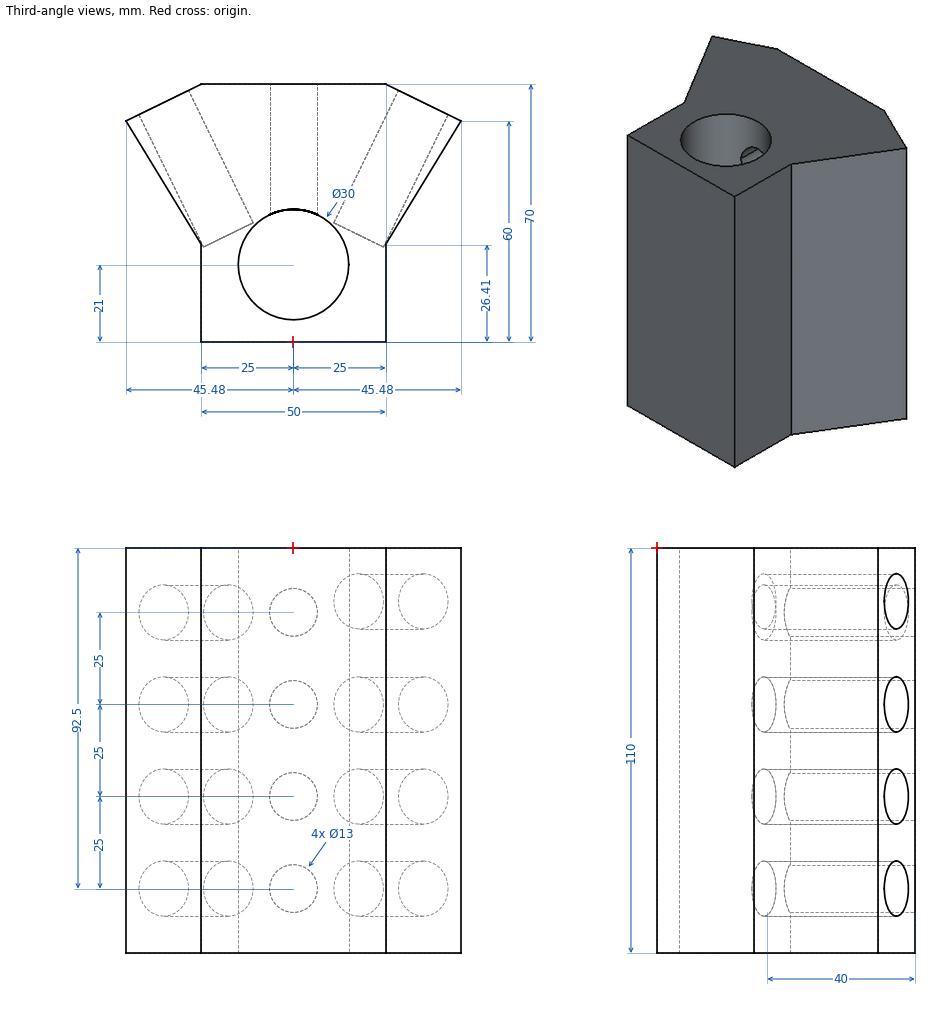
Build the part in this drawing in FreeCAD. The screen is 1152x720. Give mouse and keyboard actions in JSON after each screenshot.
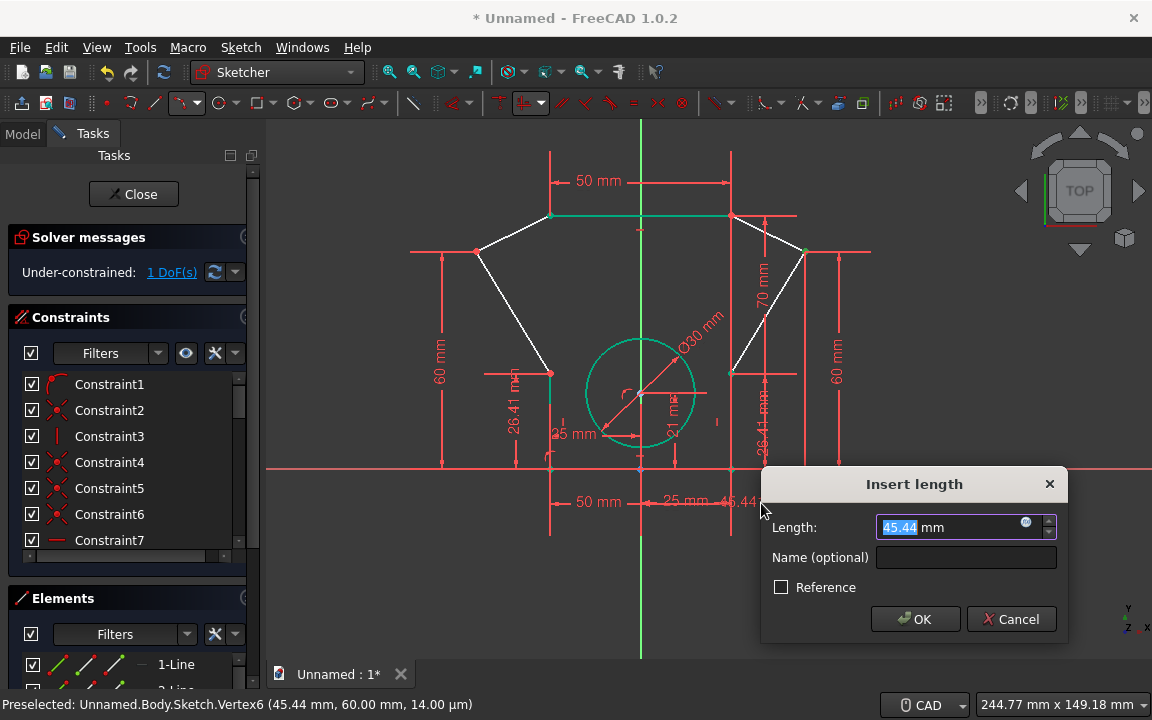
{"action": "type", "text": "45.48"}
{"action": "key", "text": "Return"}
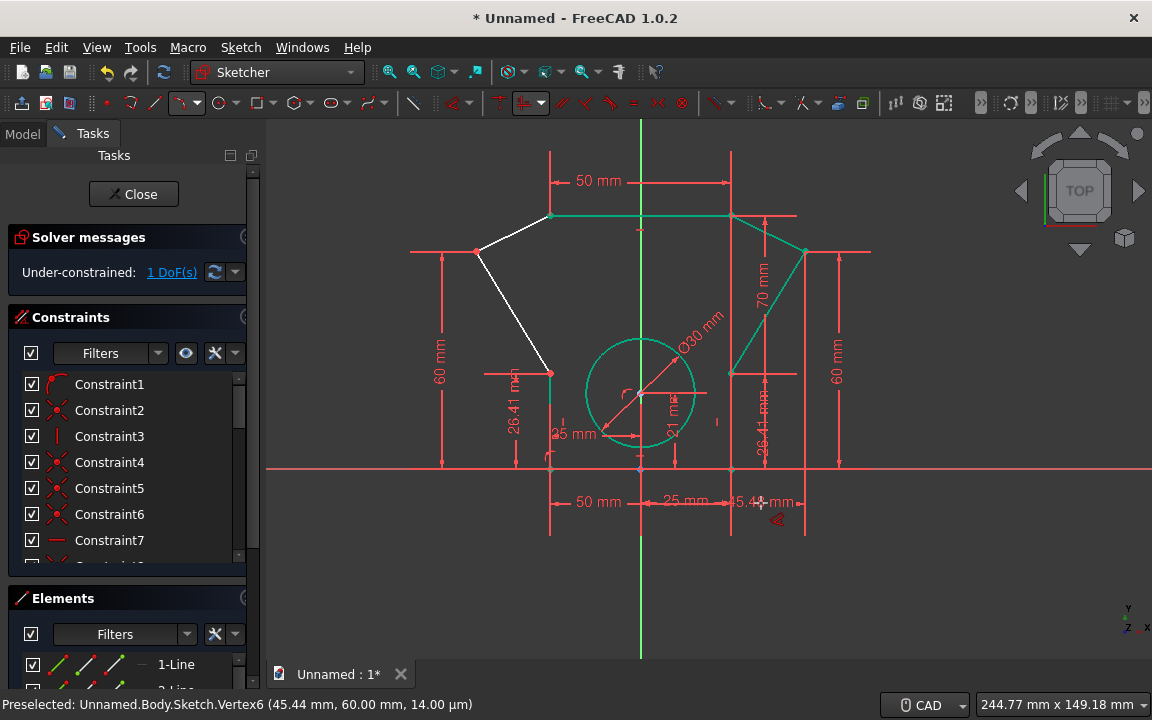
{"action": "left_click", "coordinate": [476, 252]}
{"action": "left_click", "coordinate": [520, 503]}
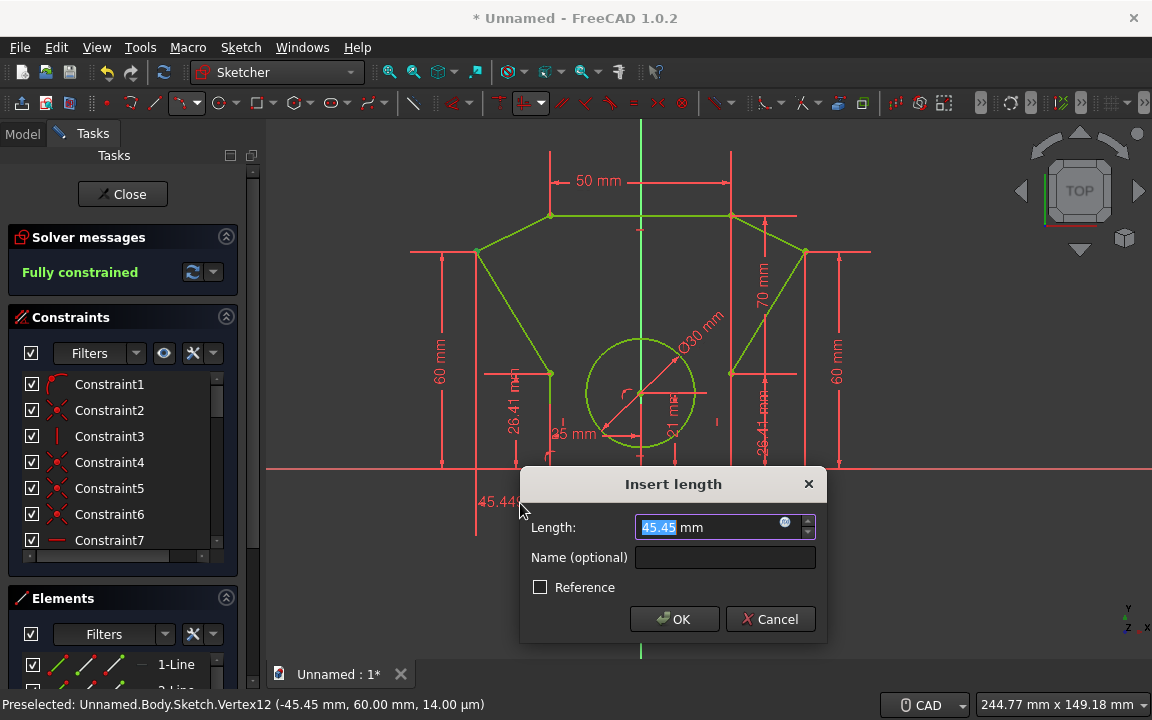
{"action": "type", "text": "45.48"}
{"action": "key", "text": "Return"}
{"action": "key", "text": "Escape"}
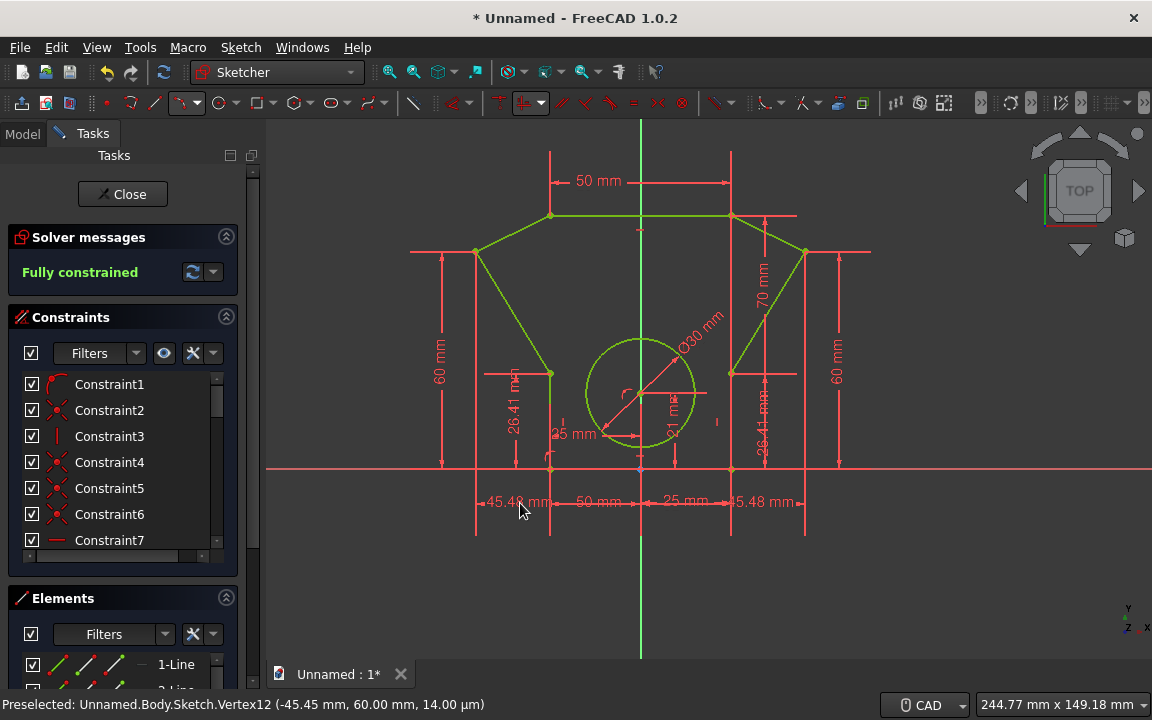
{"action": "left_click", "coordinate": [123, 194]}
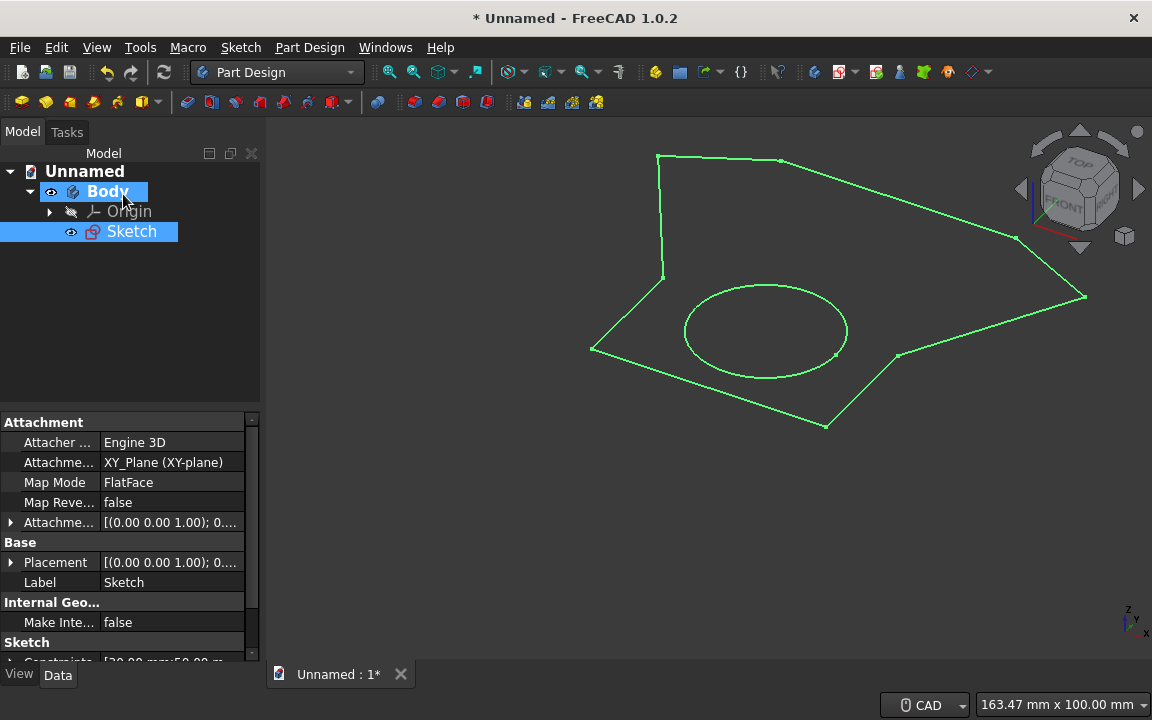
{"action": "left_click", "coordinate": [22, 102]}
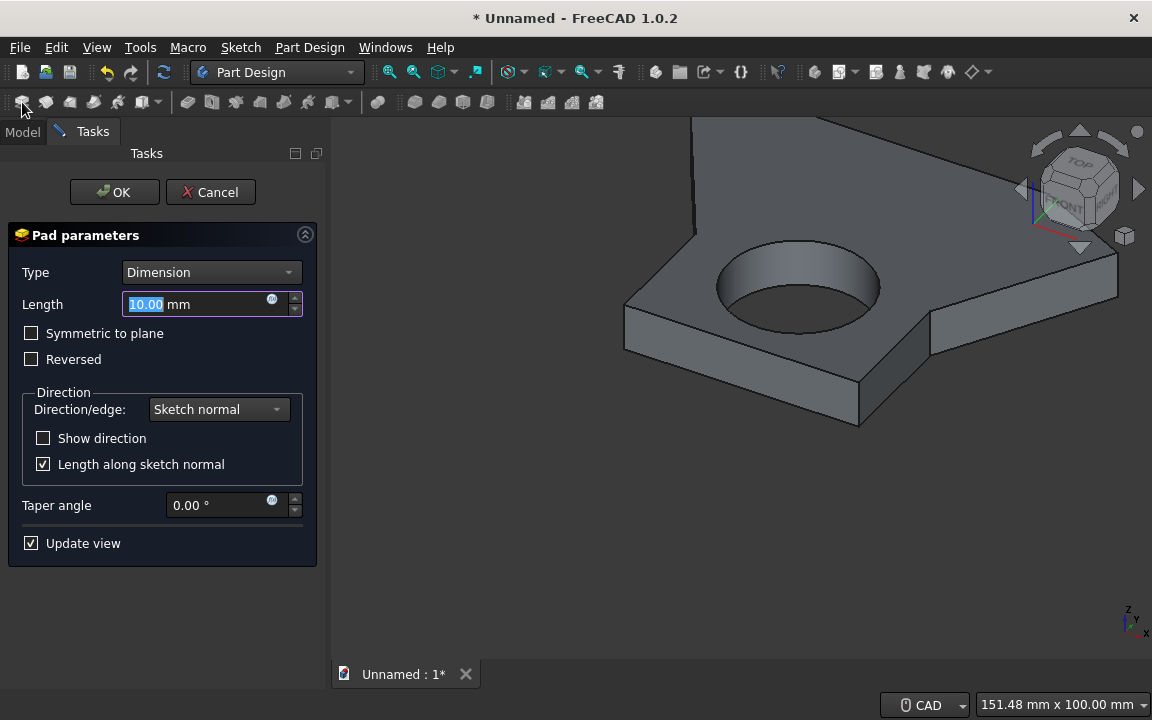
{"action": "type", "text": "110"}
{"action": "key", "text": "Tab"}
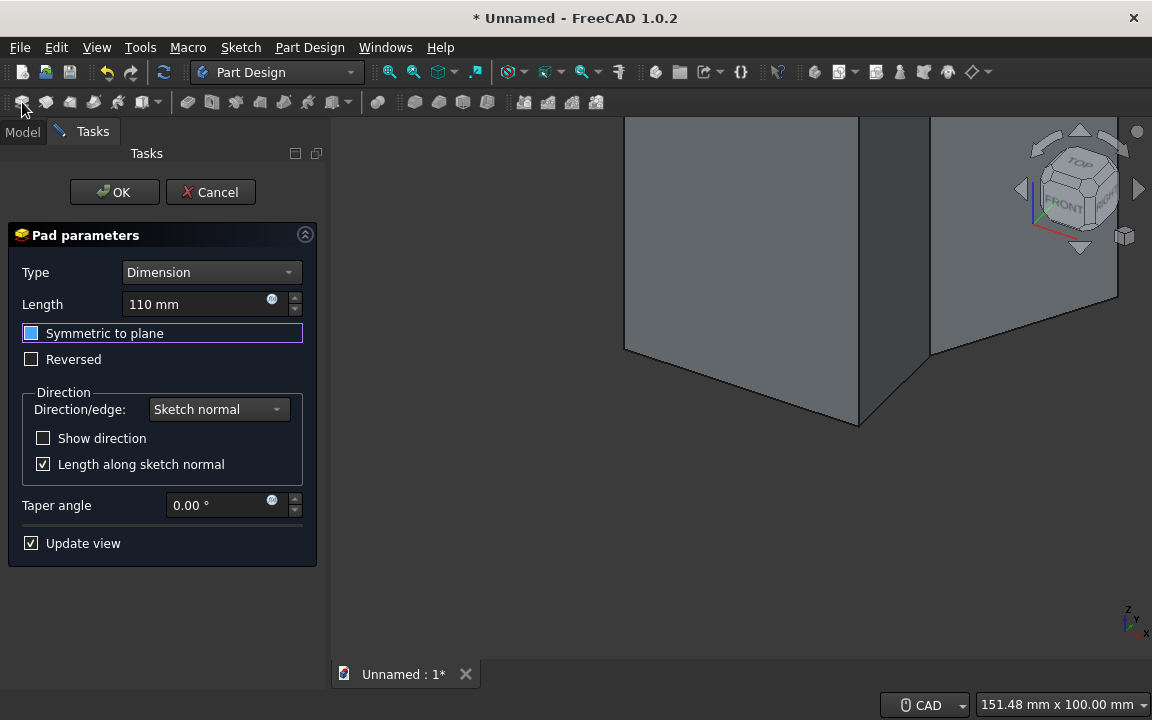
{"action": "left_click", "coordinate": [30, 359]}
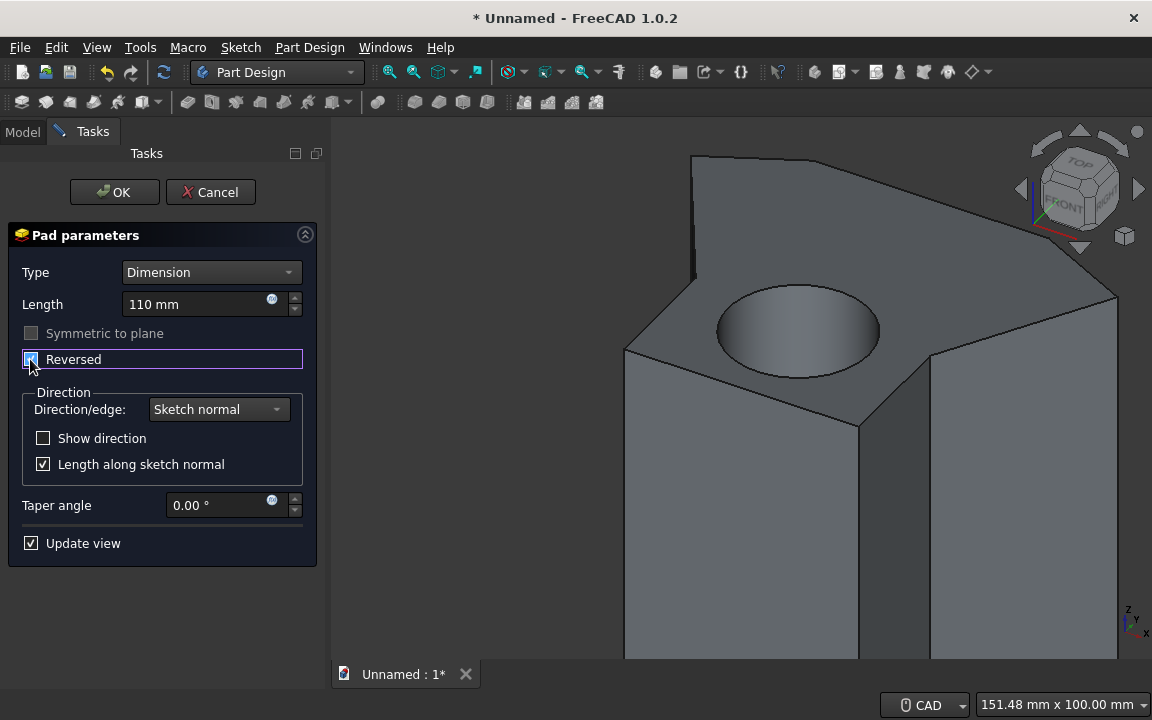
{"action": "left_click", "coordinate": [115, 192]}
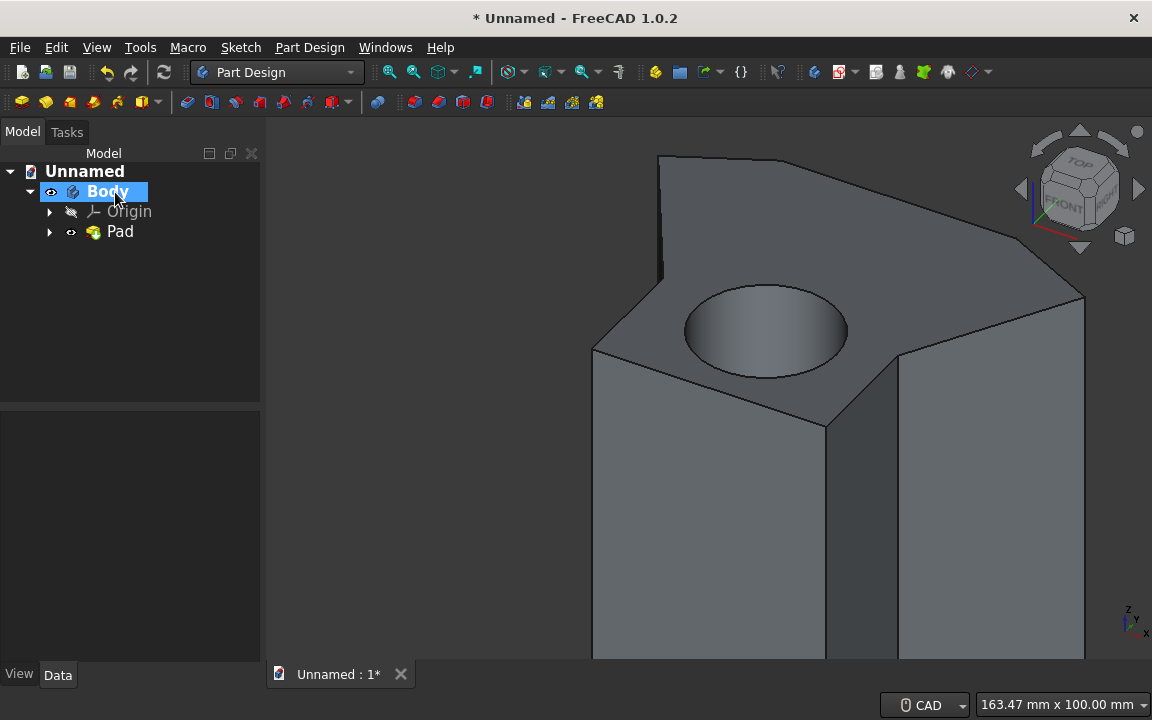
{"action": "key", "text": "v f"}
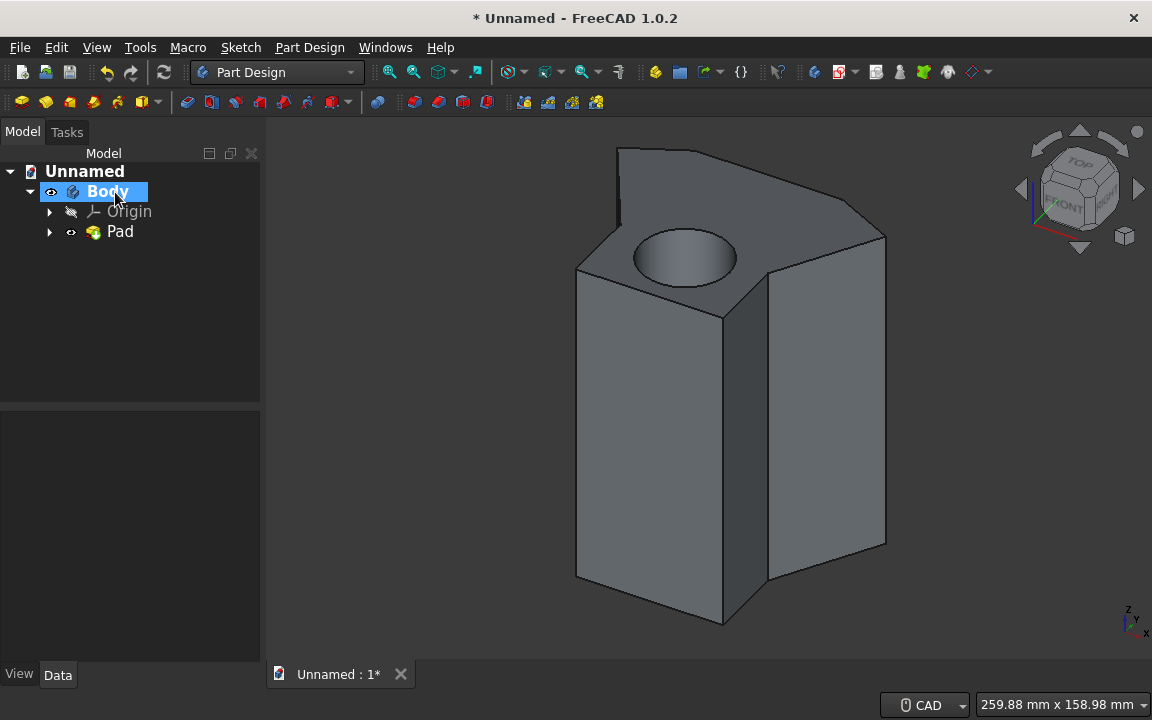
{"action": "key", "text": "4"}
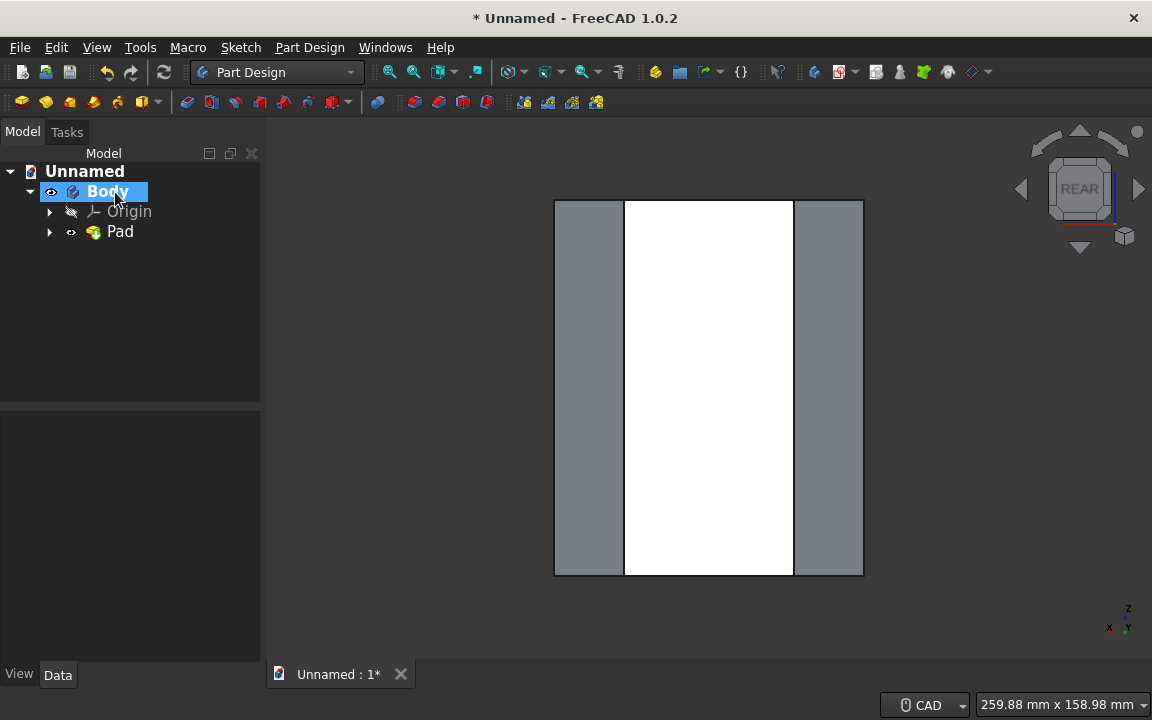
{"action": "left_click", "coordinate": [589, 280]}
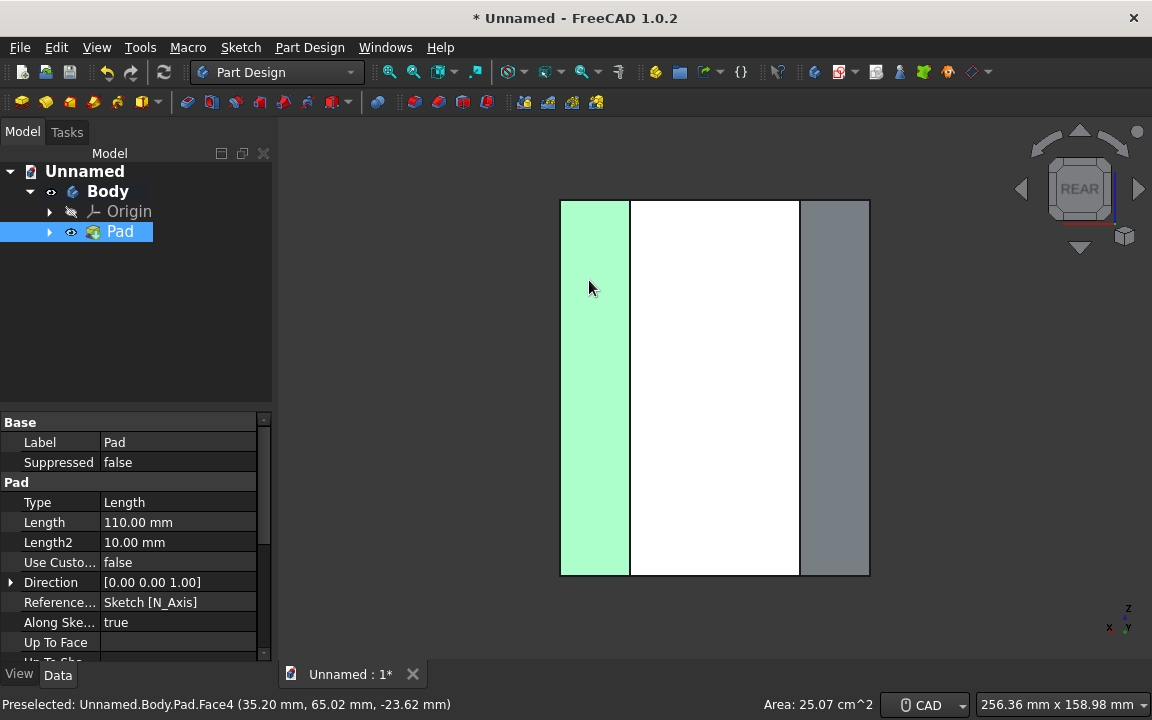
{"action": "left_click", "coordinate": [840, 72]}